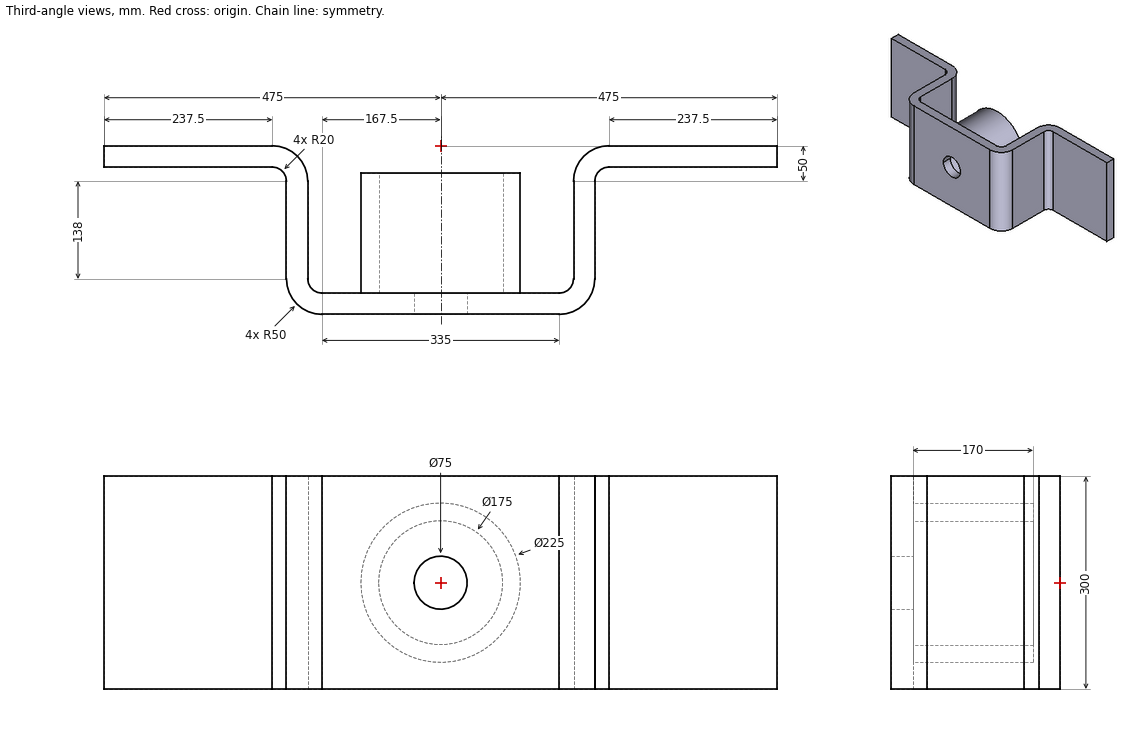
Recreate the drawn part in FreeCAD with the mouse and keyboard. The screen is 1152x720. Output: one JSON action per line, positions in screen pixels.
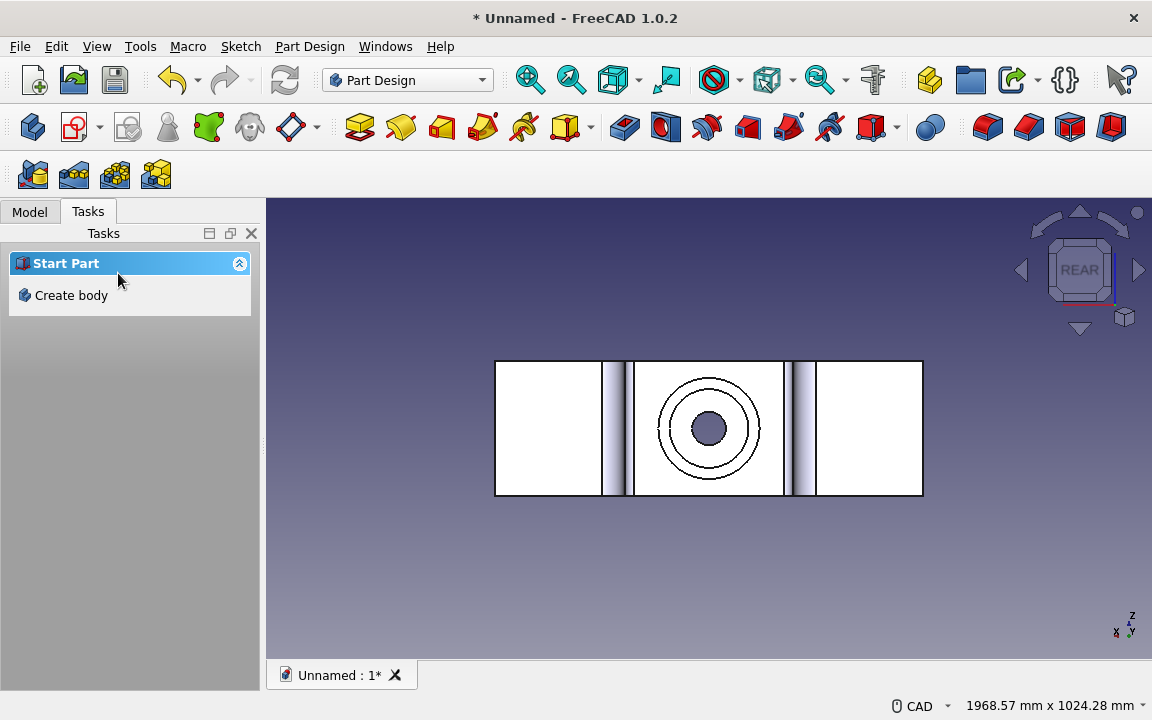
{"action": "key", "text": "0"}